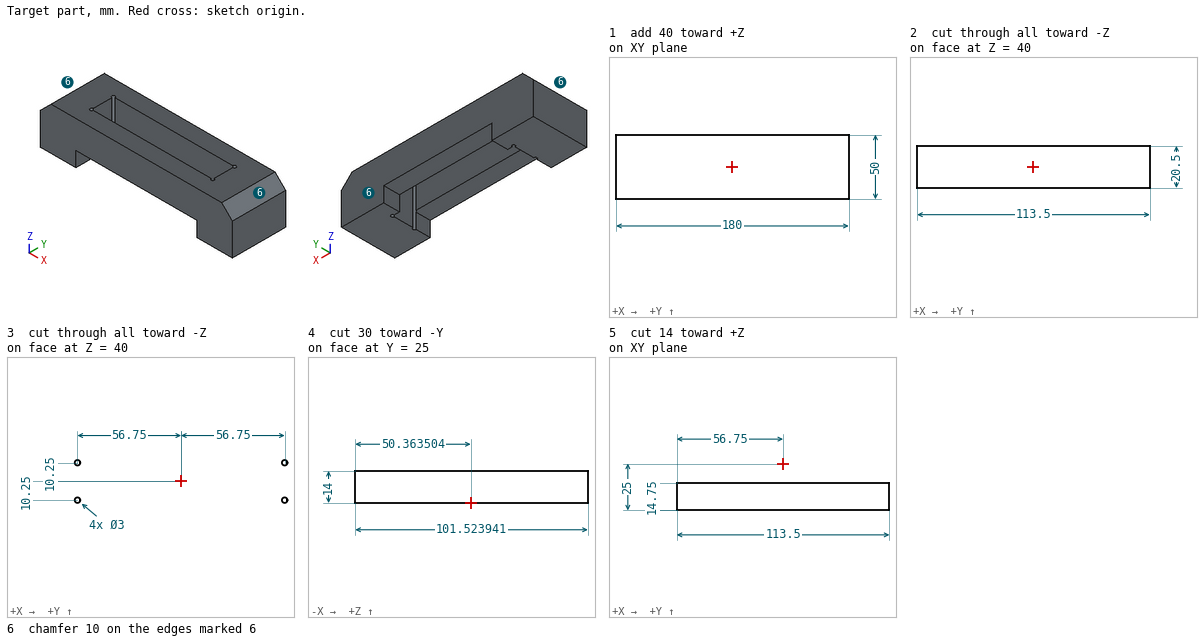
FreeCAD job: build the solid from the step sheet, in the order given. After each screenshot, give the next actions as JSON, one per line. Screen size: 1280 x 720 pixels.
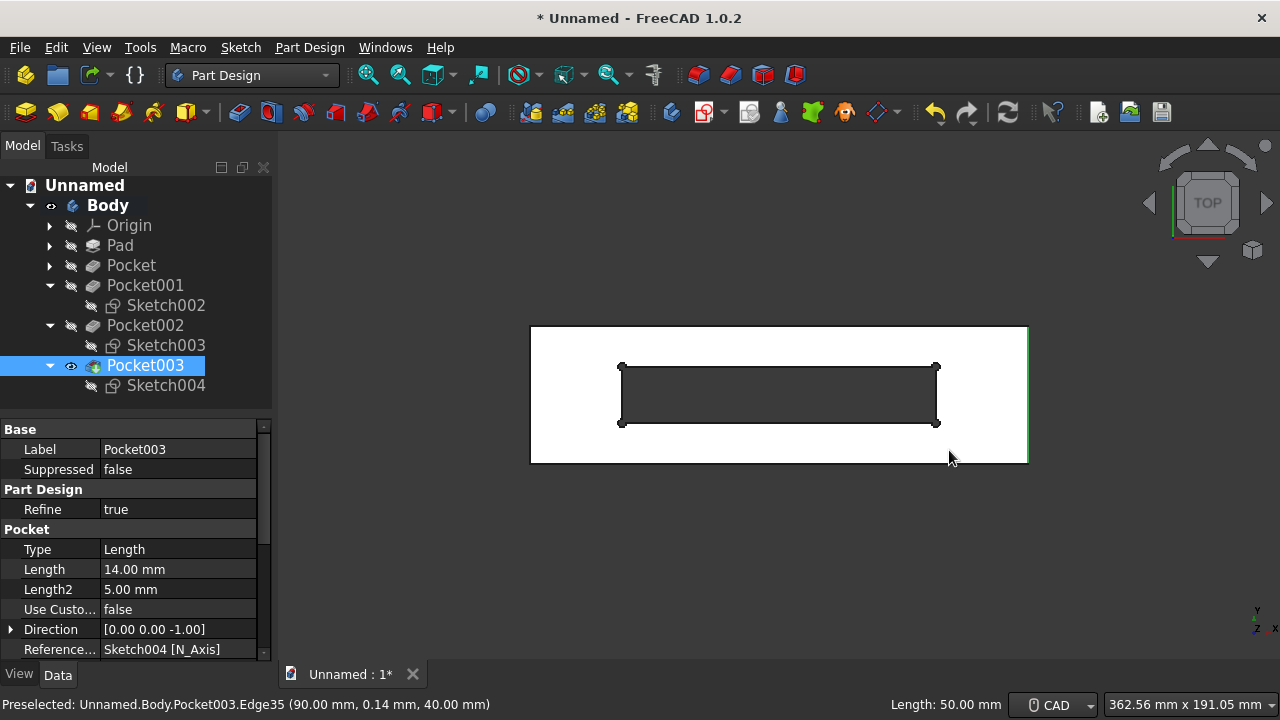
{"action": "left_click", "coordinate": [530, 394], "text": "ctrl"}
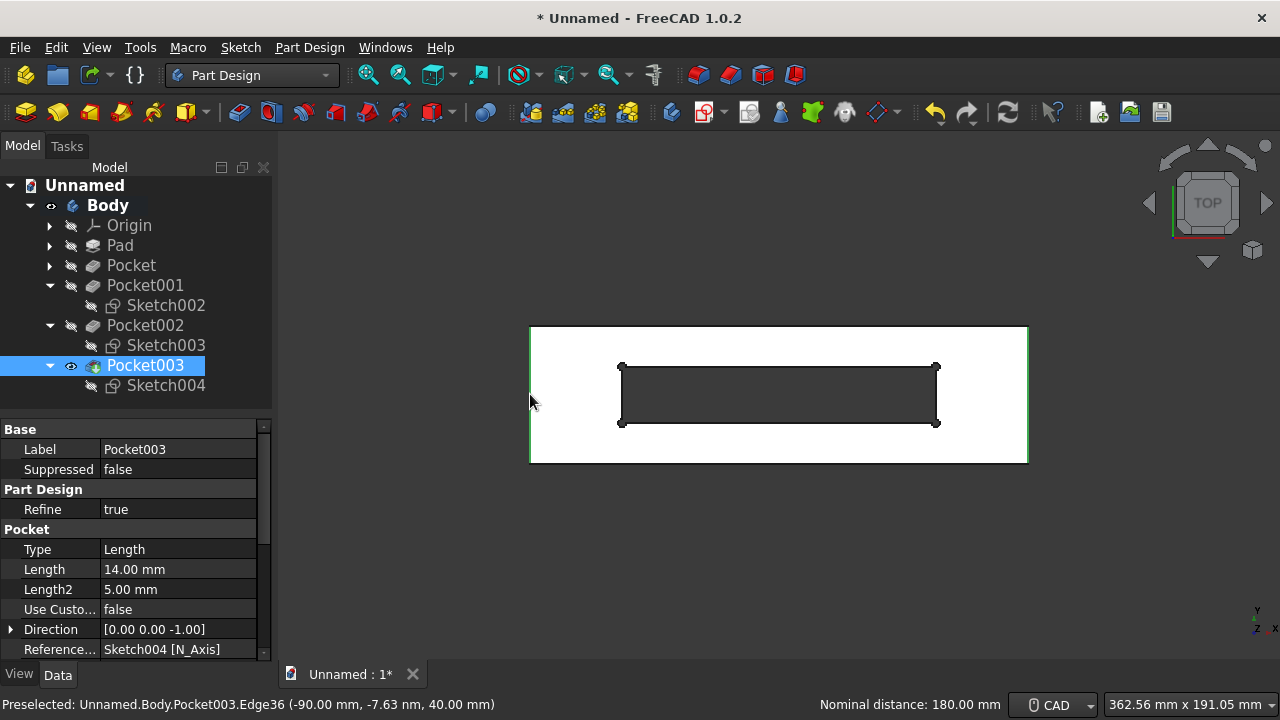
{"action": "left_click", "coordinate": [732, 76]}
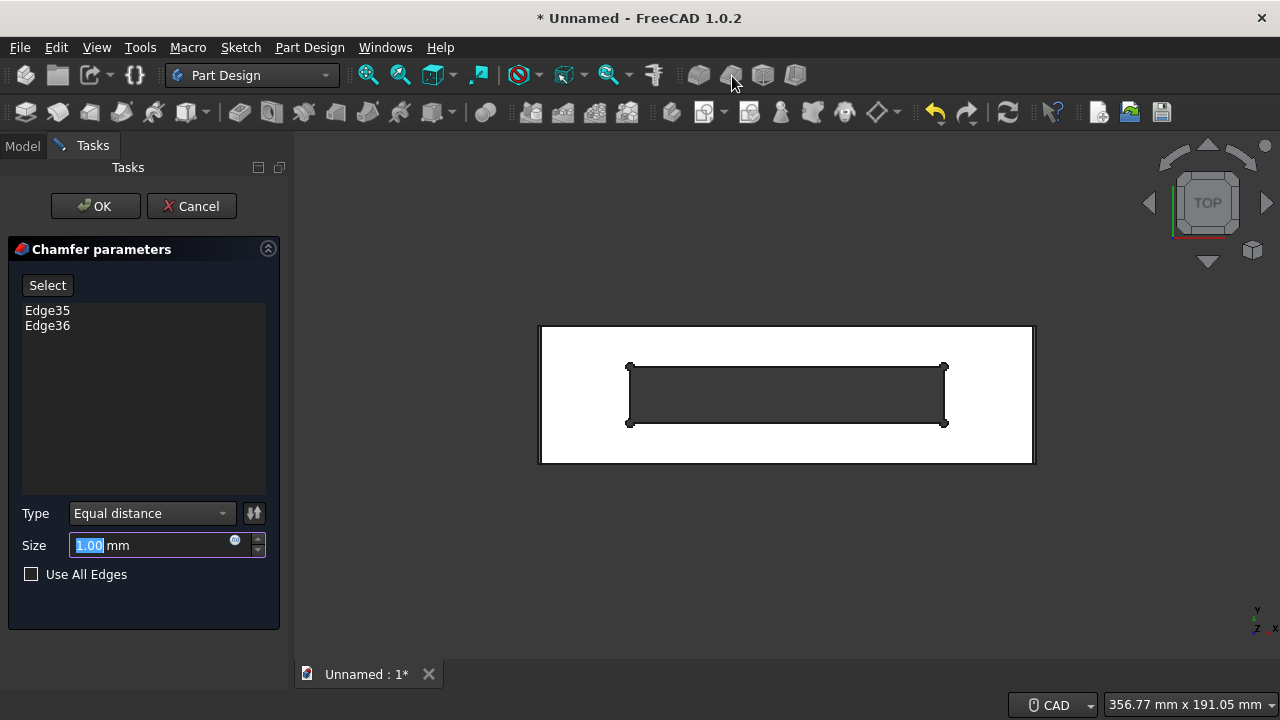
{"action": "type", "text": "10"}
{"action": "key", "text": "Tab"}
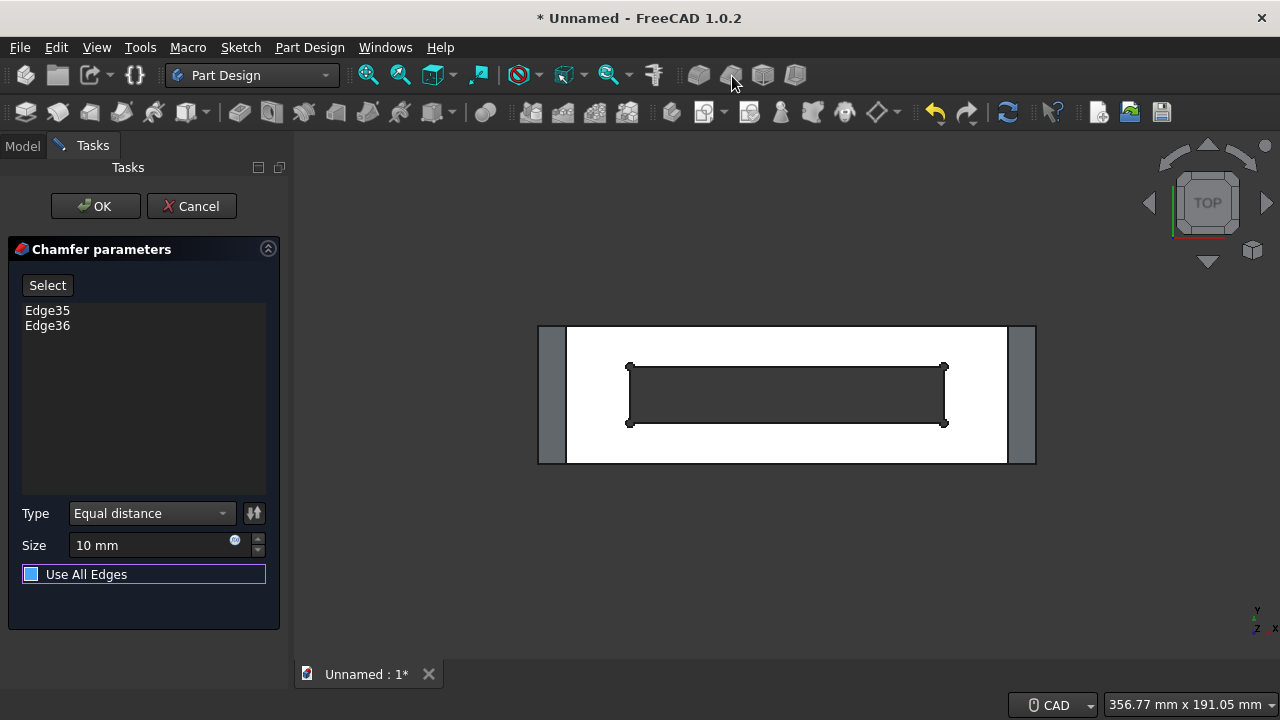
{"action": "left_click", "coordinate": [96, 206]}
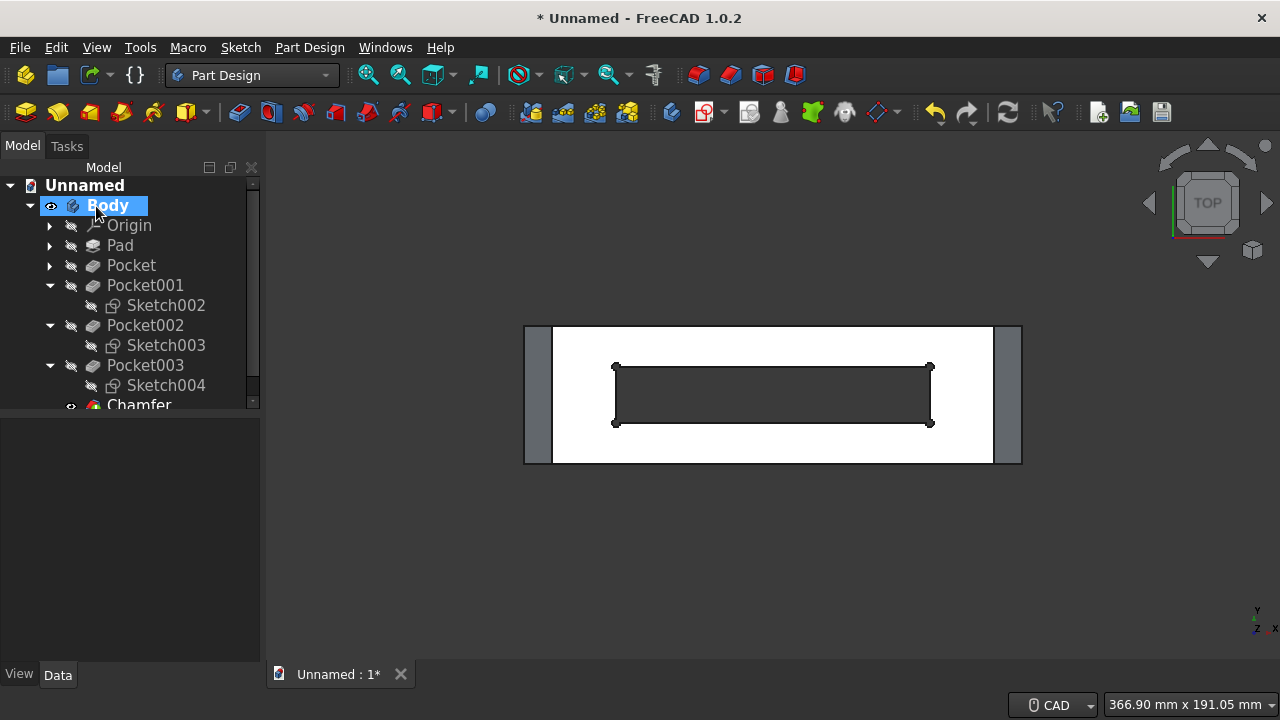
{"action": "key", "text": "0"}